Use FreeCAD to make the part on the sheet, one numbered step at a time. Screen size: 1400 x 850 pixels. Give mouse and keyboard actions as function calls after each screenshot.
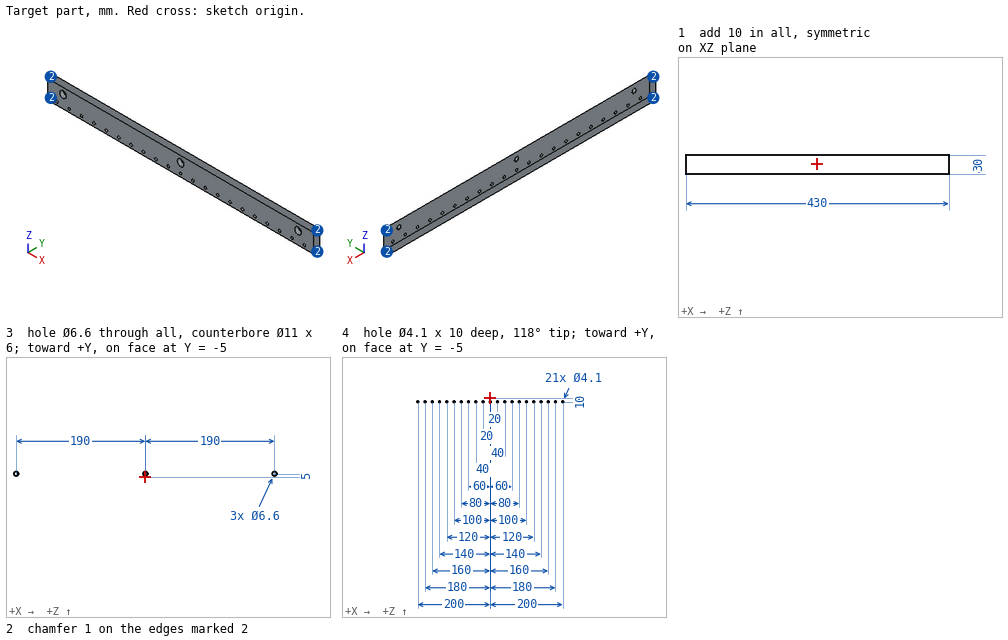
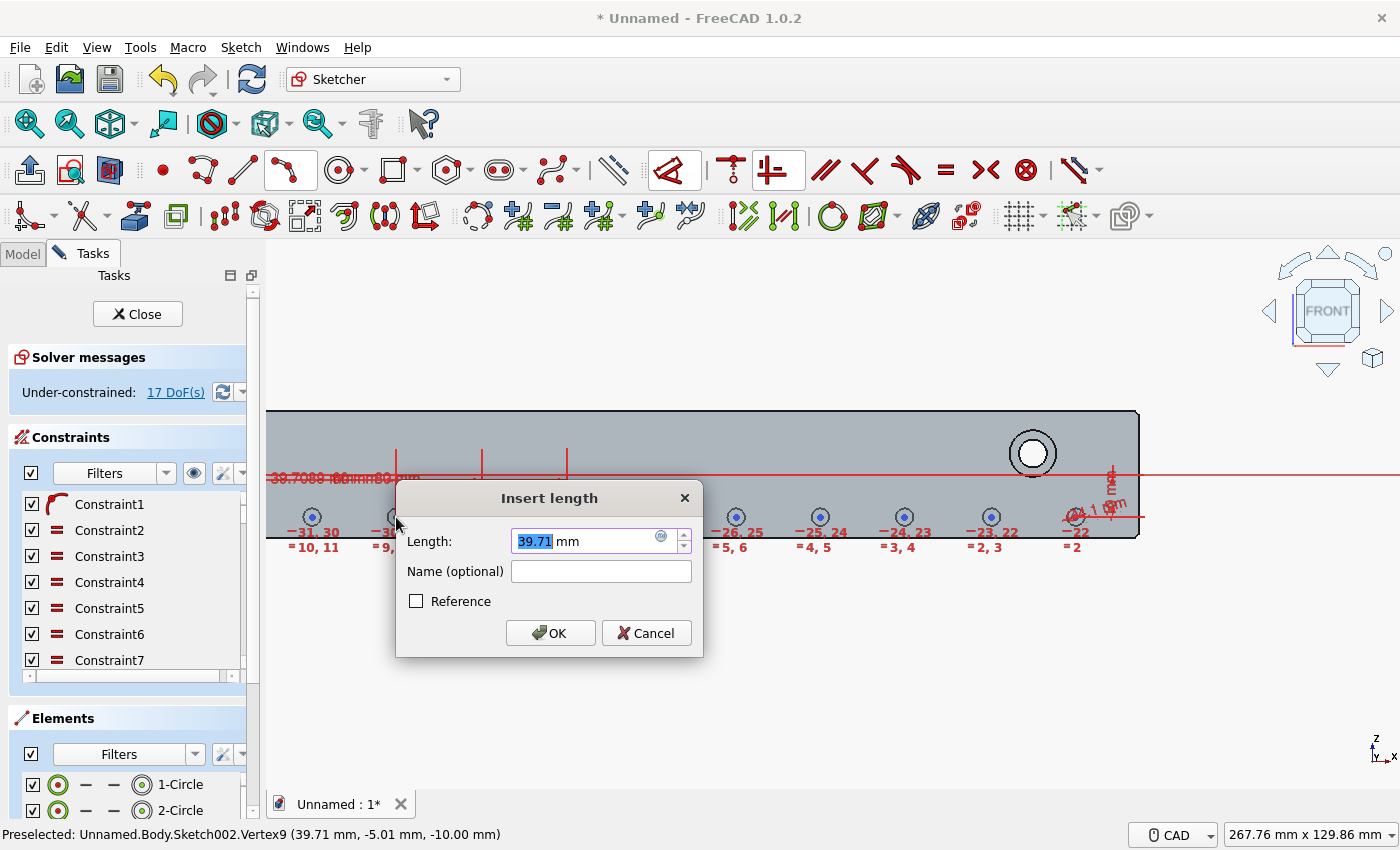
text(40)
key(Return)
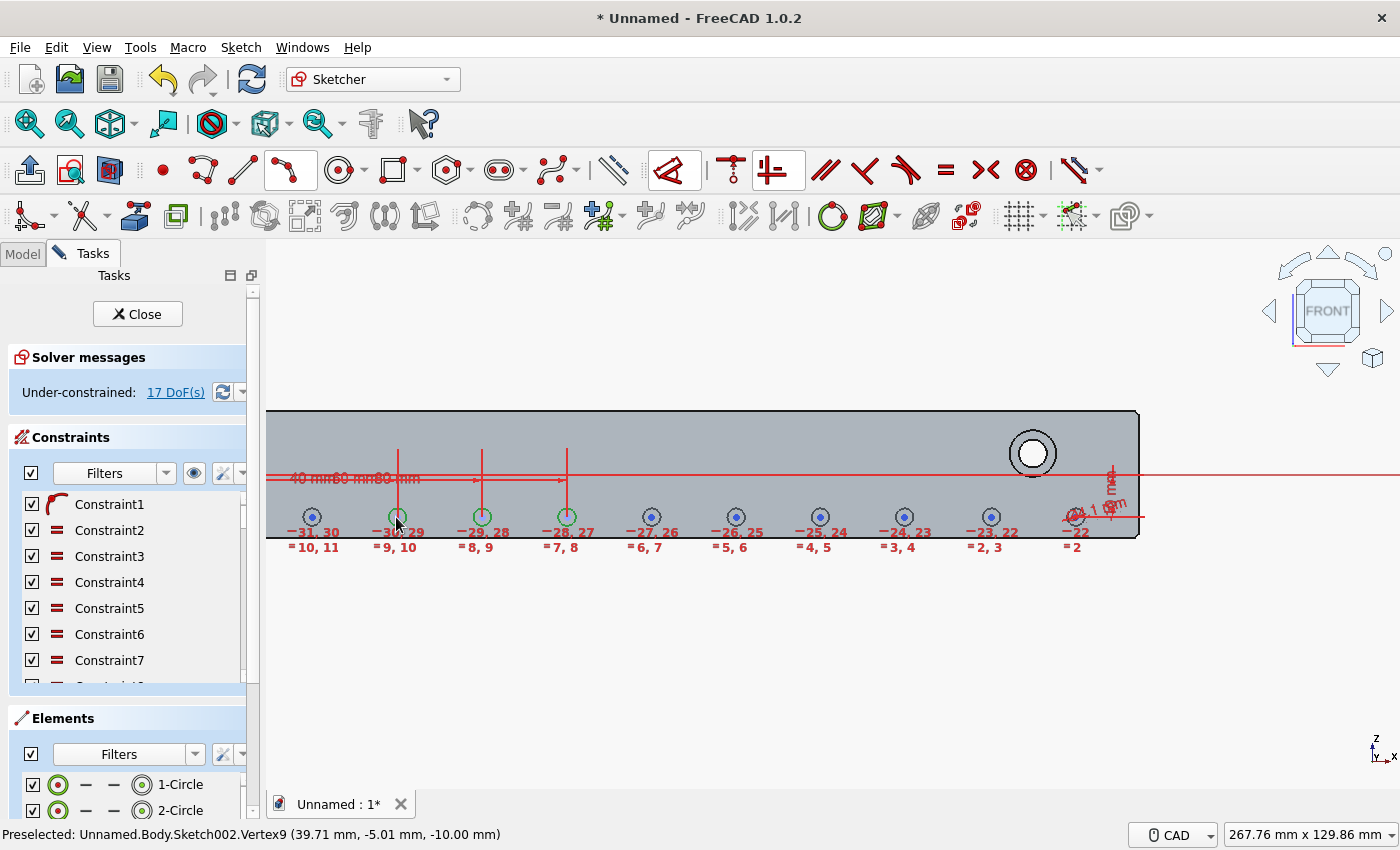
click(312, 517)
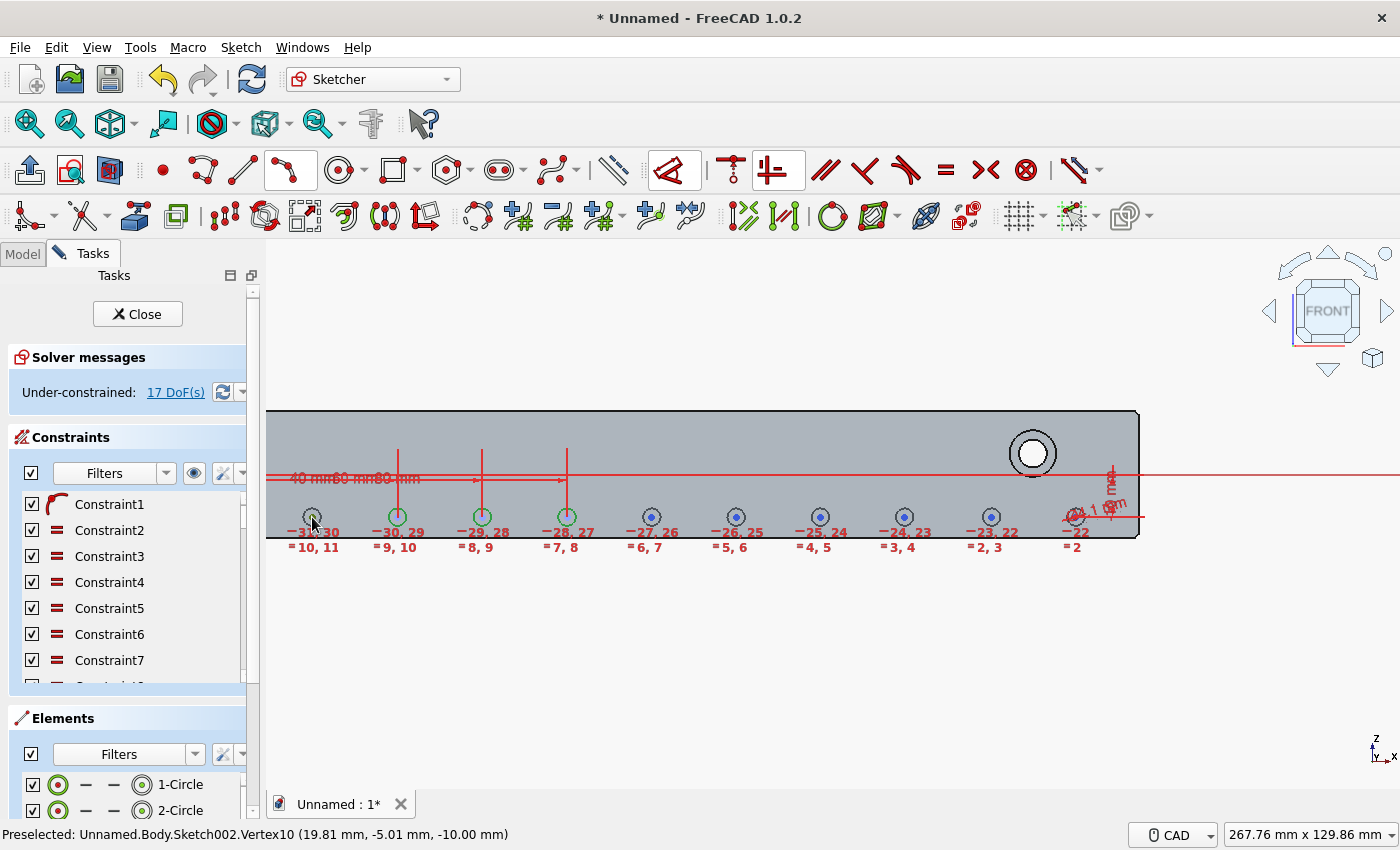
click(696, 170)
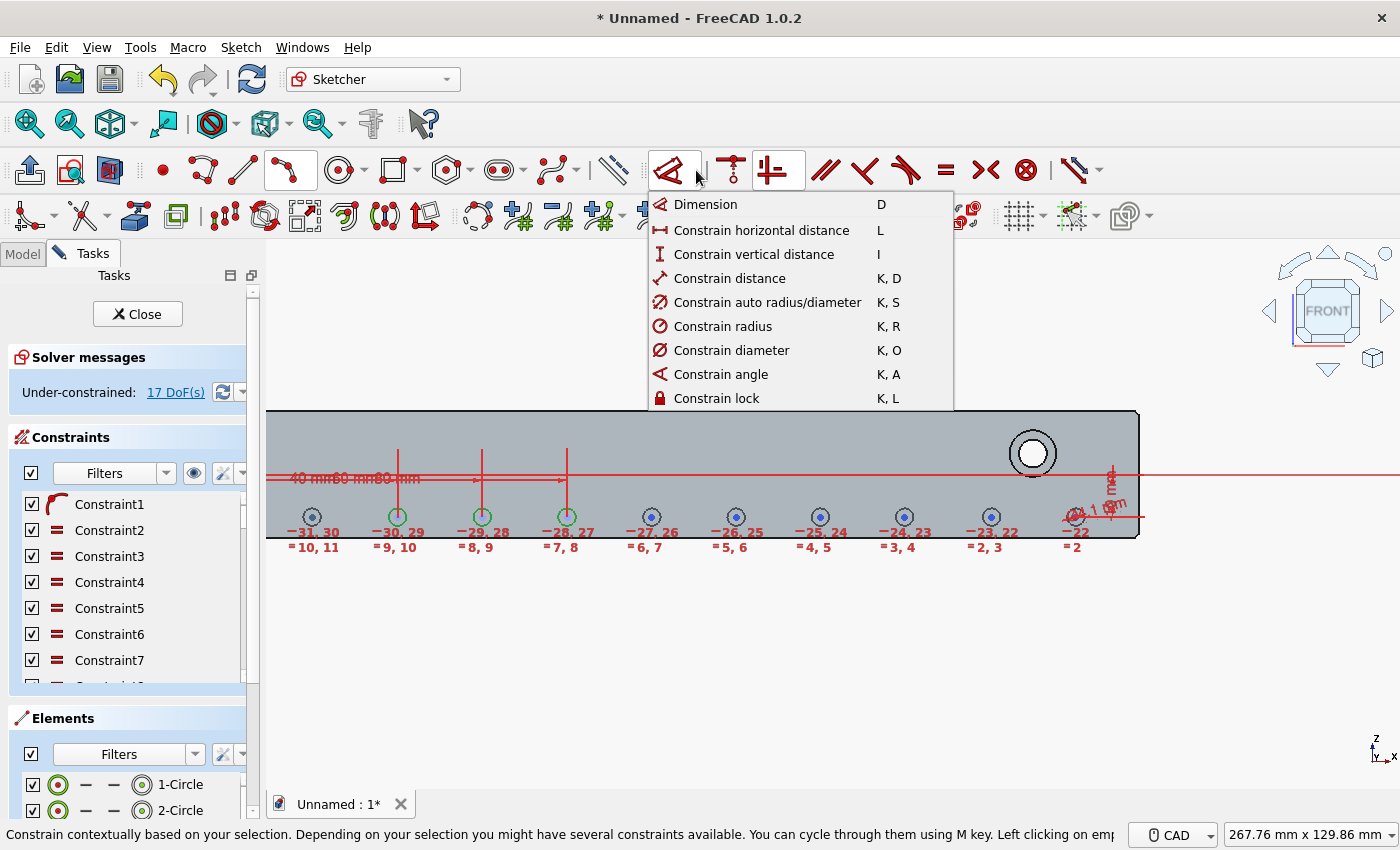
click(801, 230)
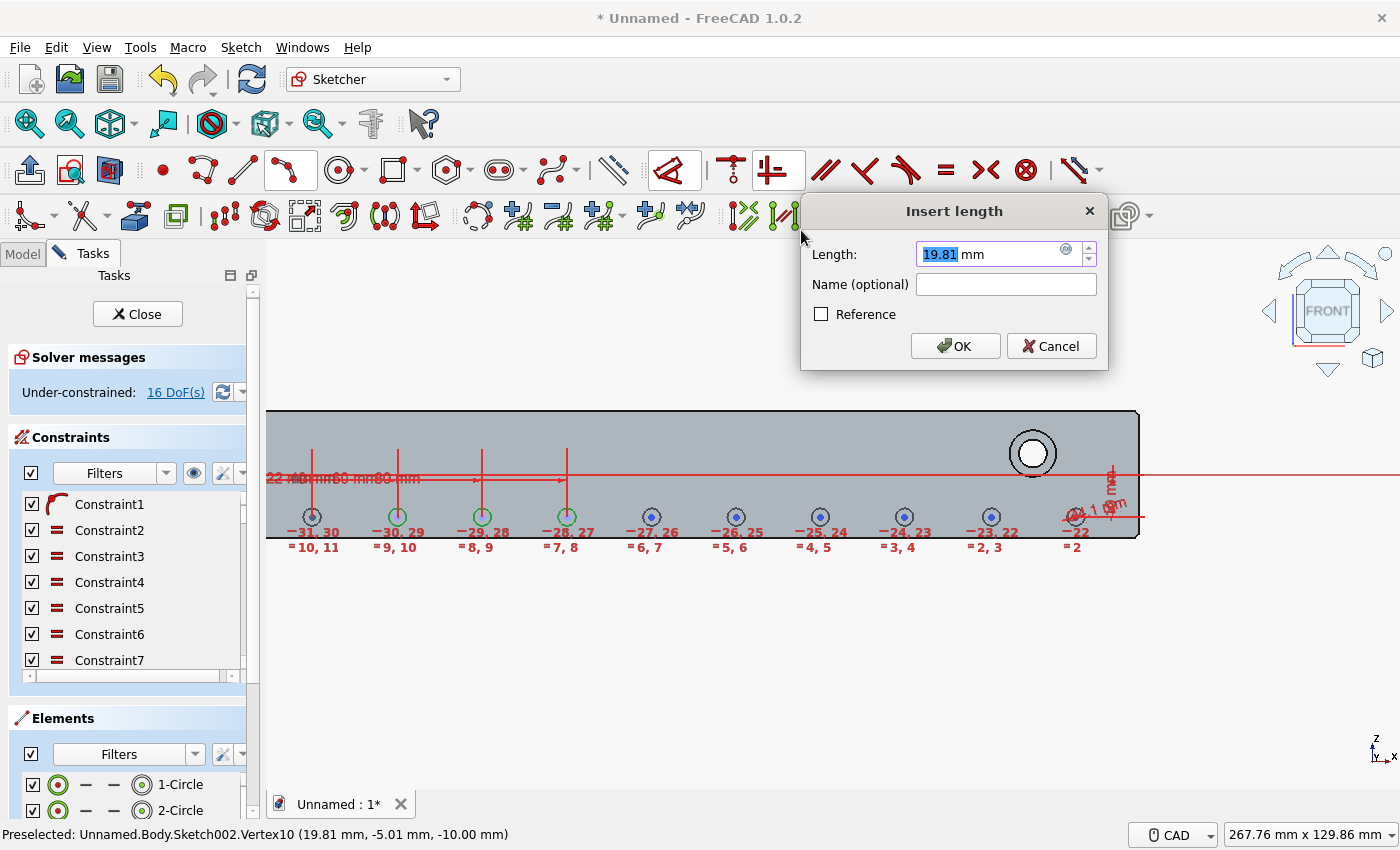
text(20)
key(Return)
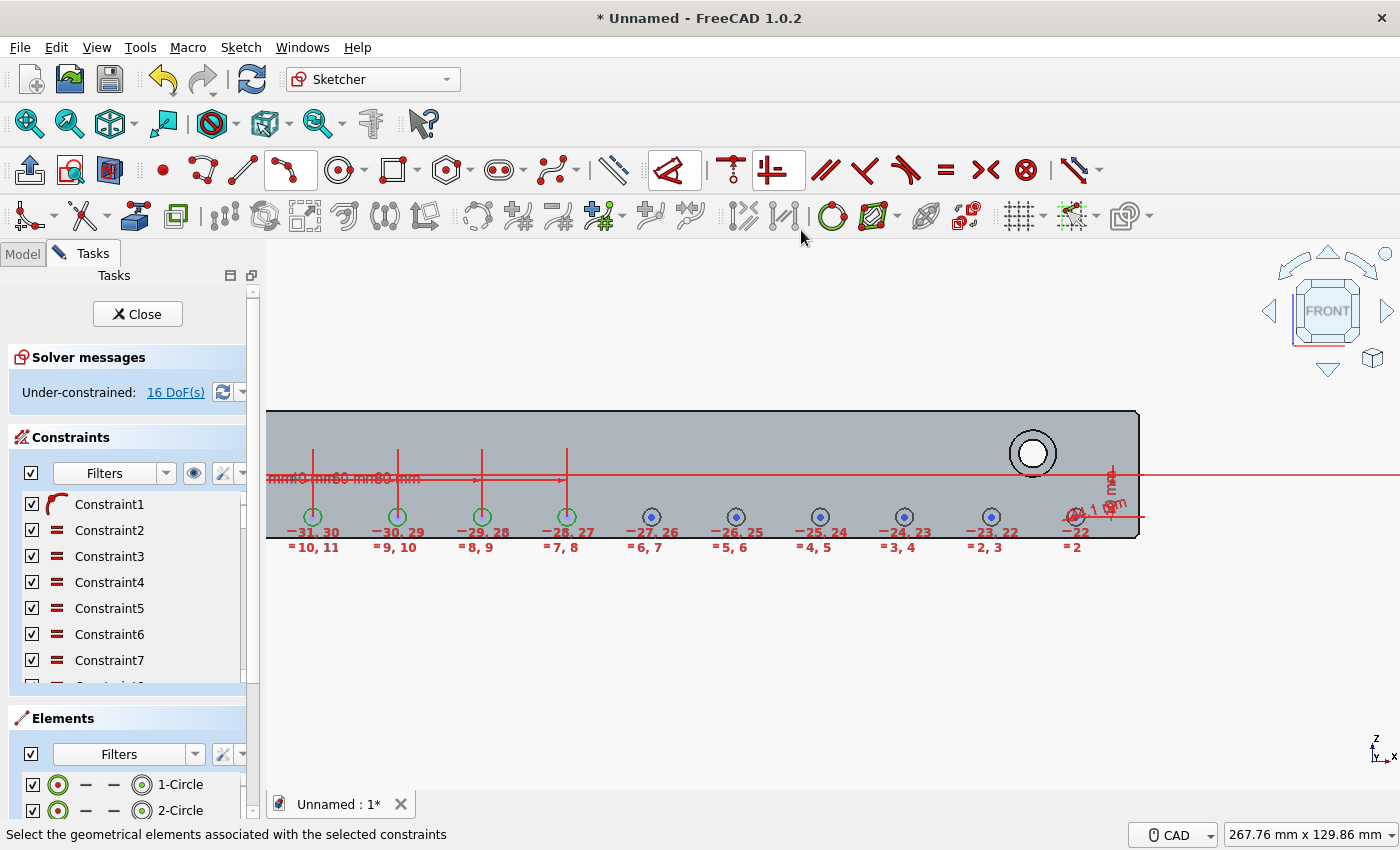
scroll(1077, 522, down, 5)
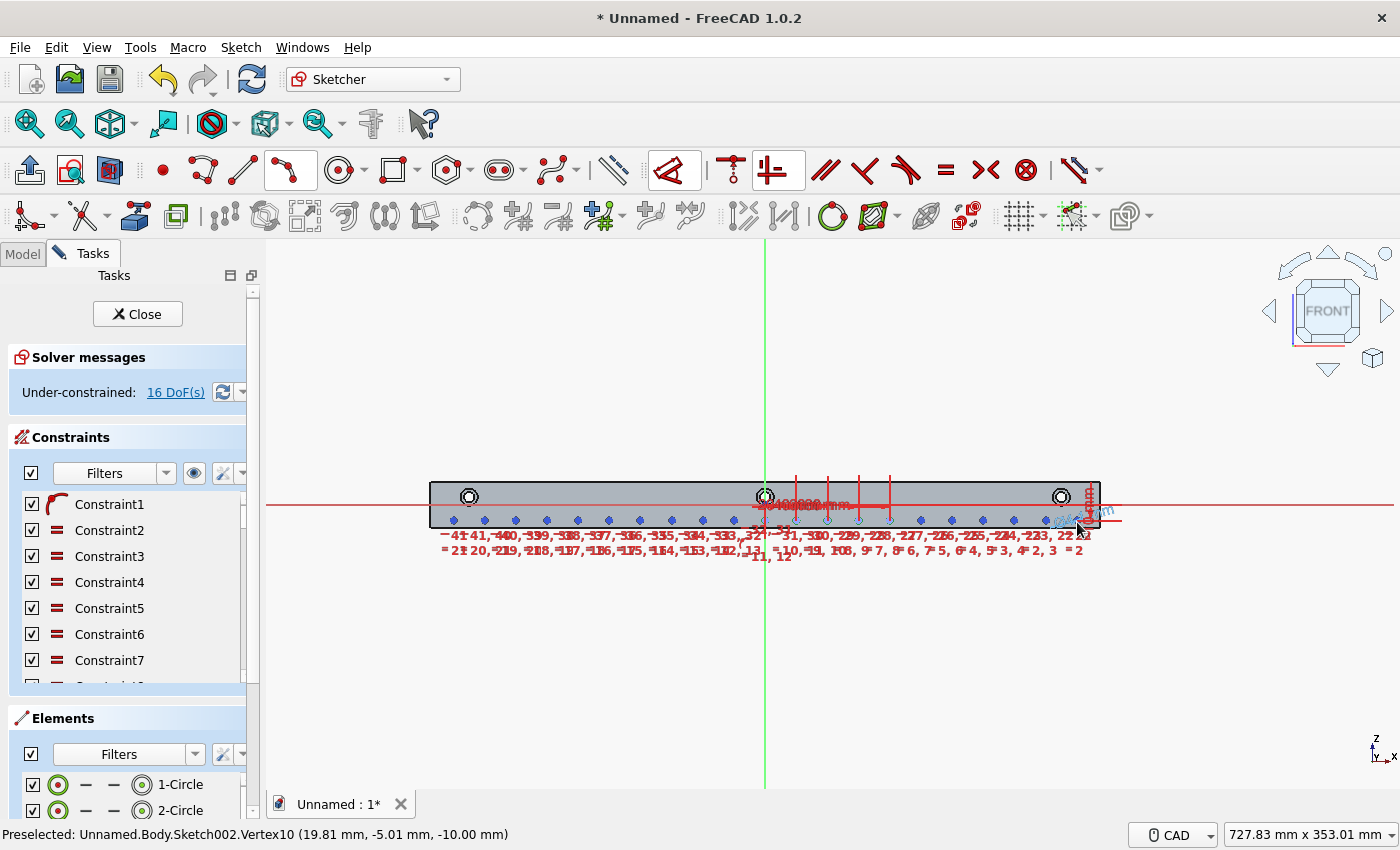
scroll(734, 521, up, 2)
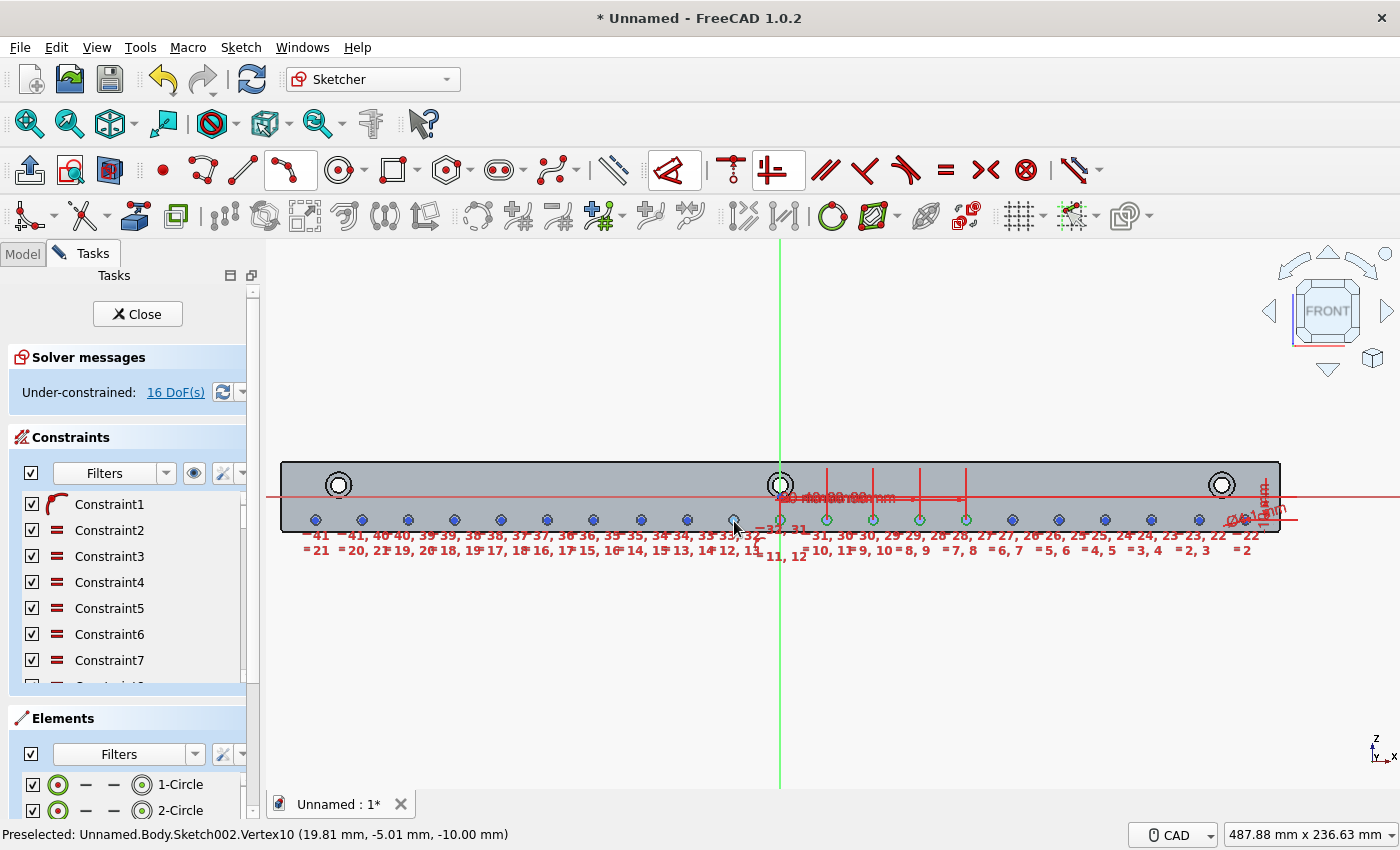
click(734, 520)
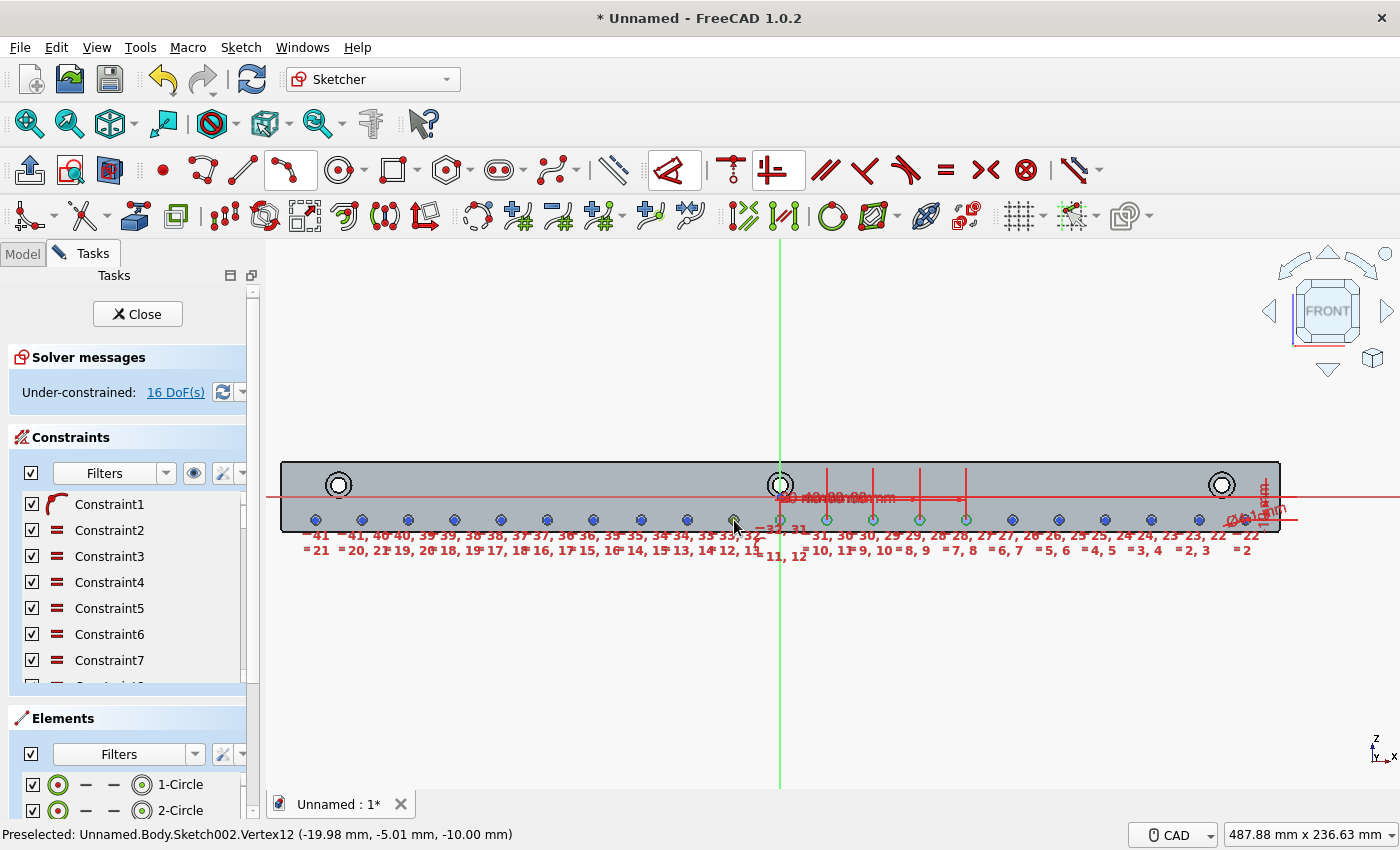
click(696, 170)